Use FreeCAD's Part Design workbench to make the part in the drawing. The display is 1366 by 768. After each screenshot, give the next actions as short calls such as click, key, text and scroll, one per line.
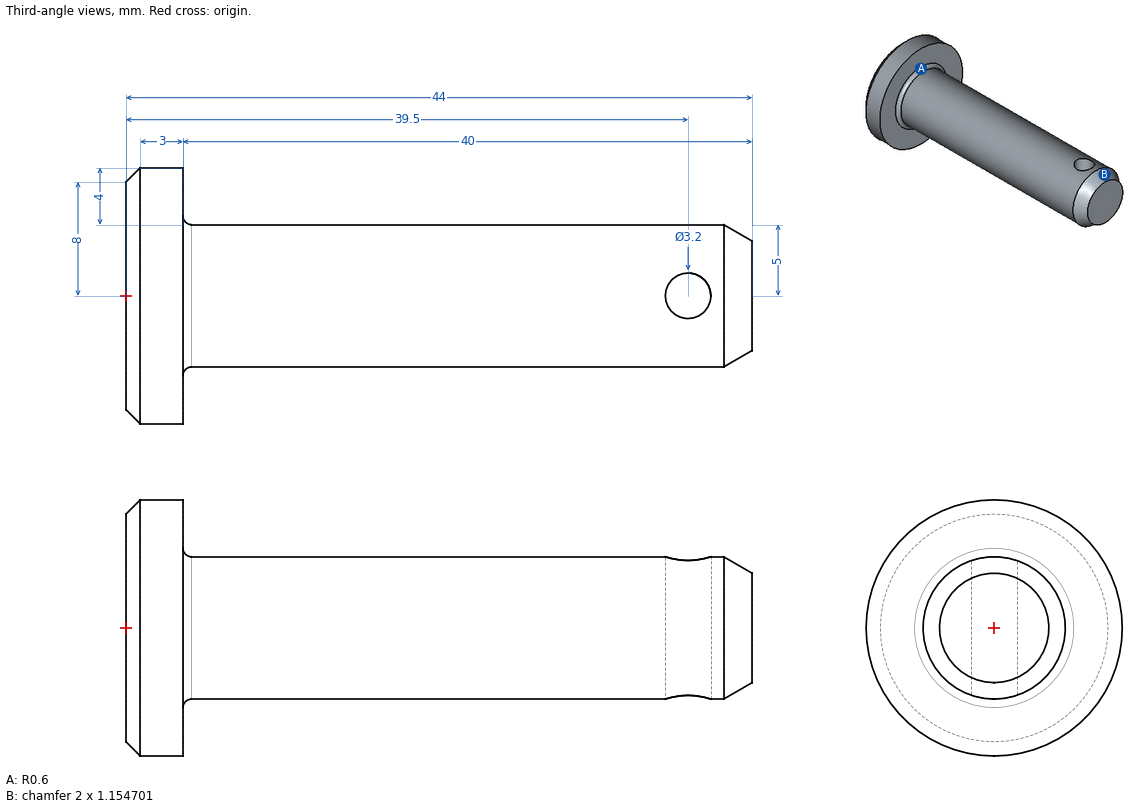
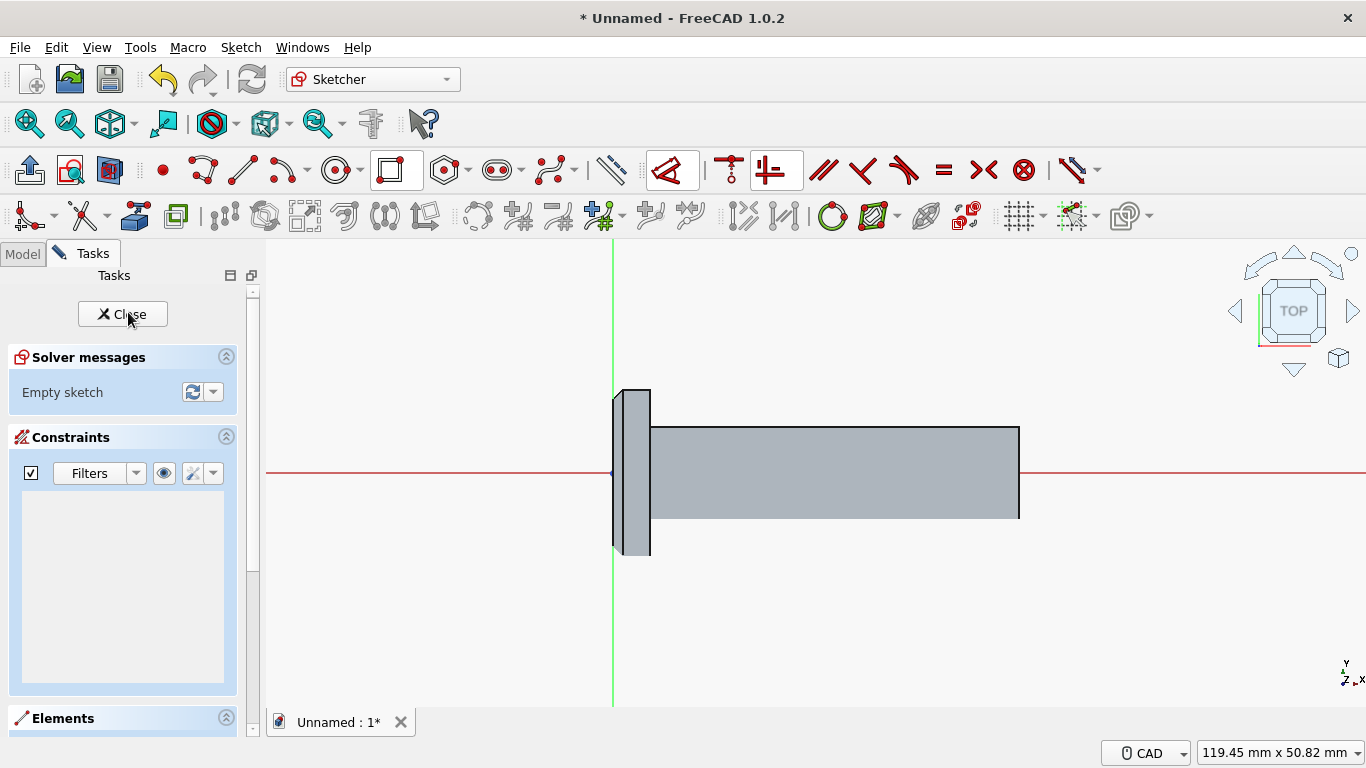
key(q)
key(s)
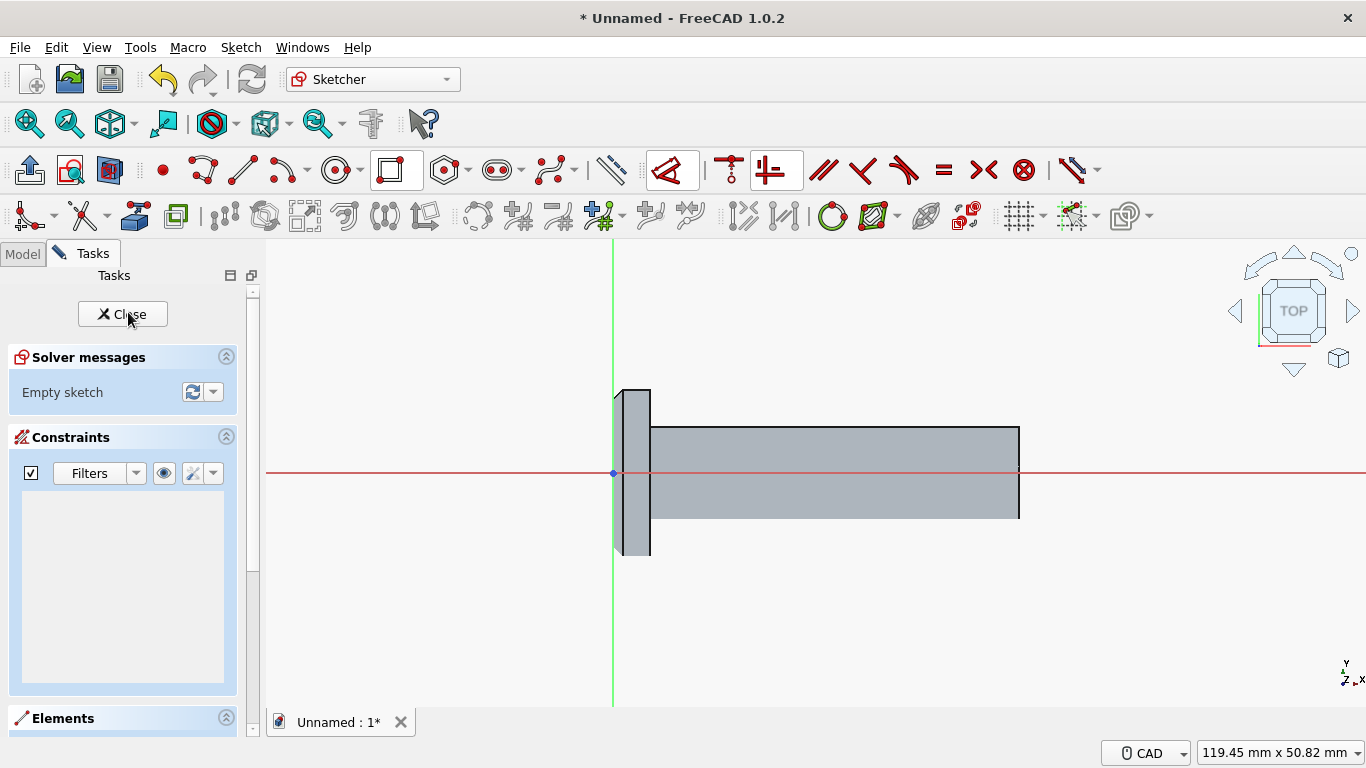
scroll(1006, 473, up, 11)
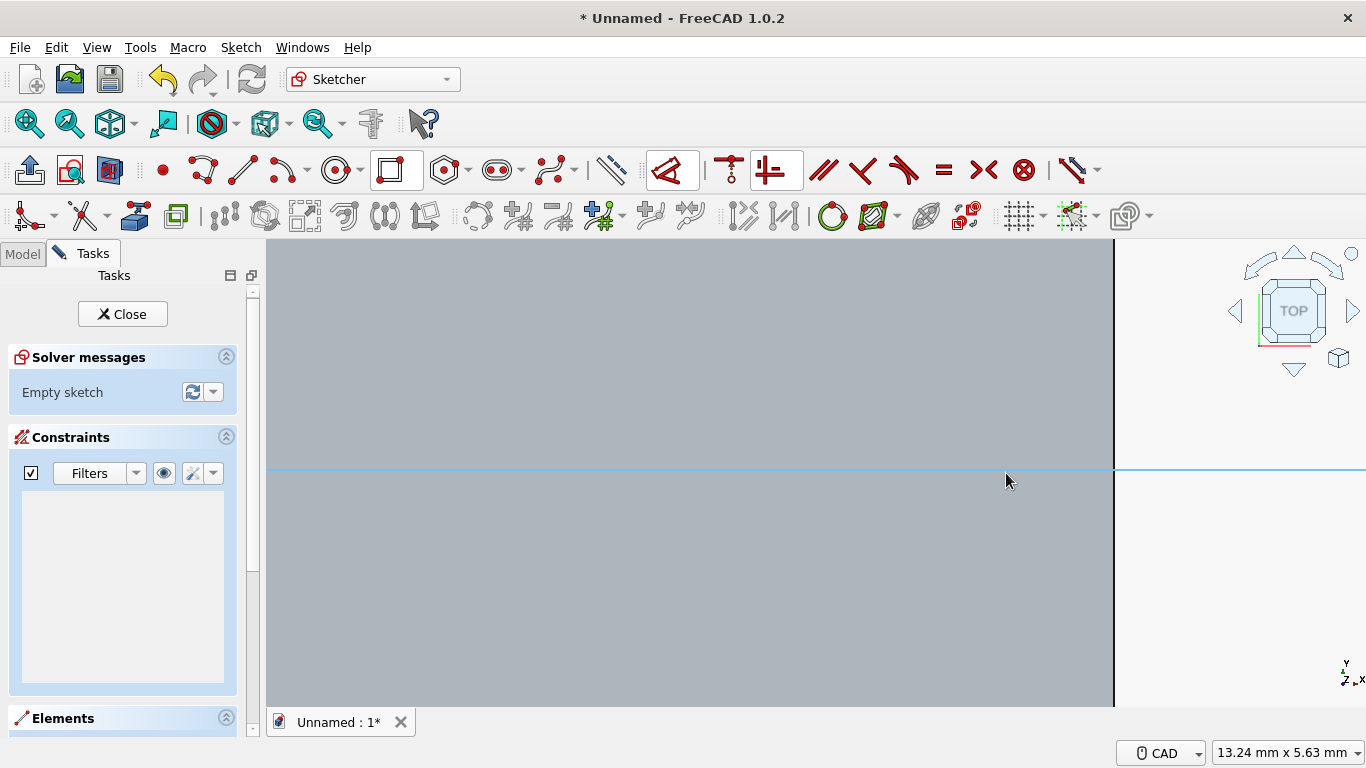
key(g)
key(c)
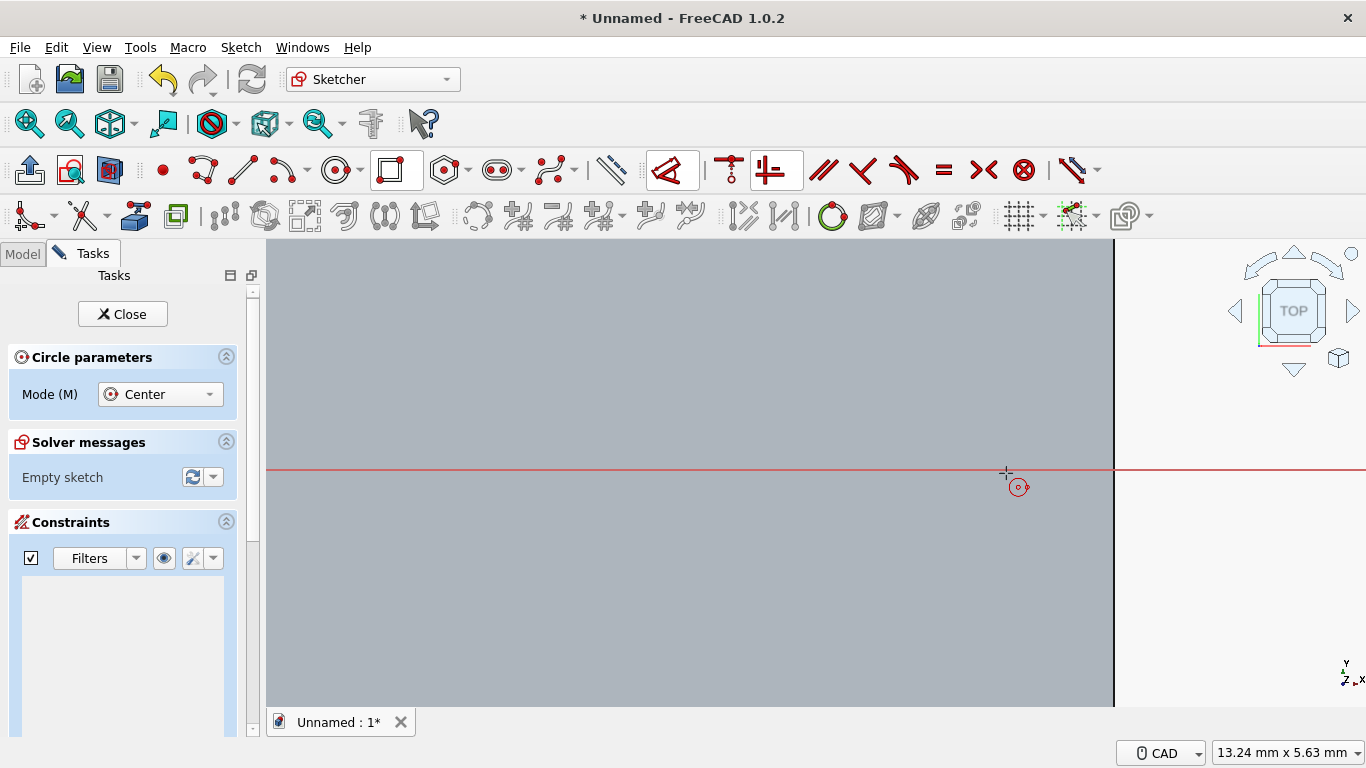
click(740, 470)
move(834, 376)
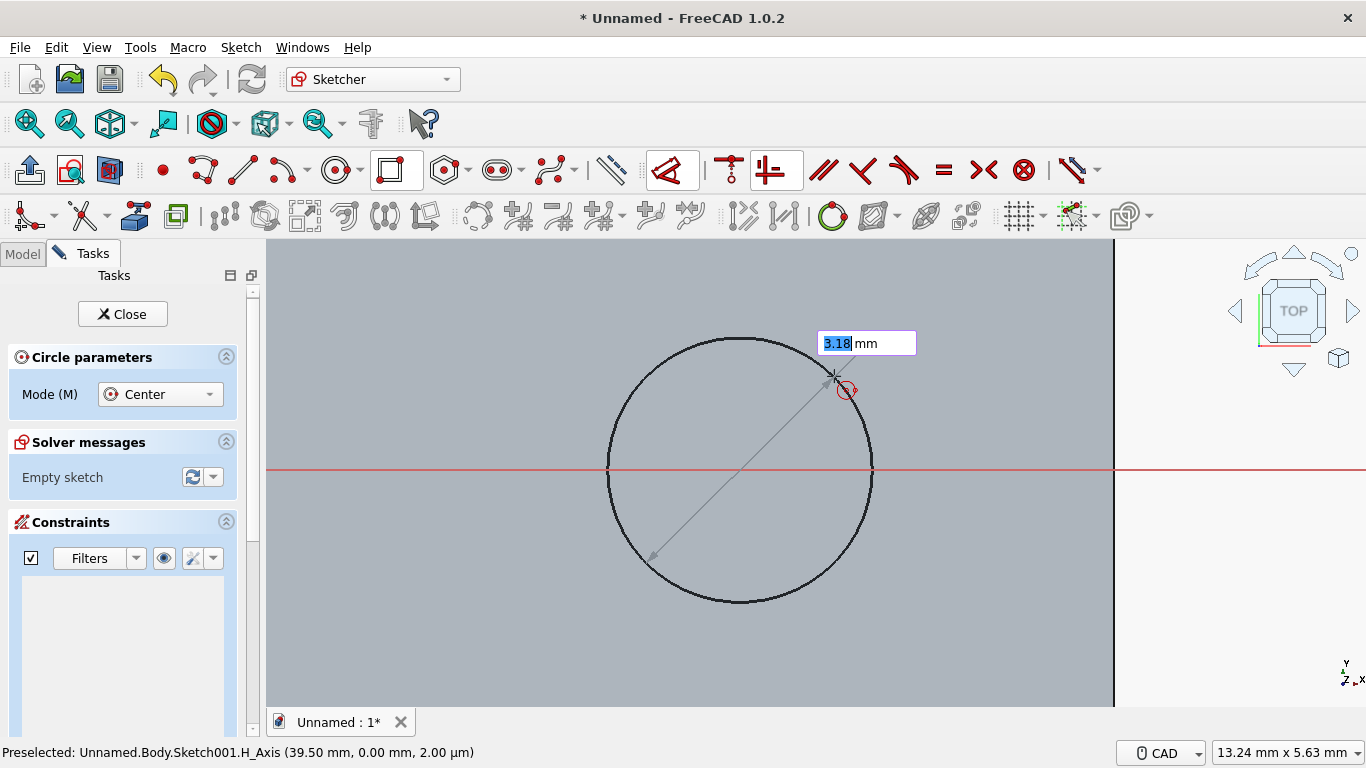
text(3.2)
key(Return)
key(Escape)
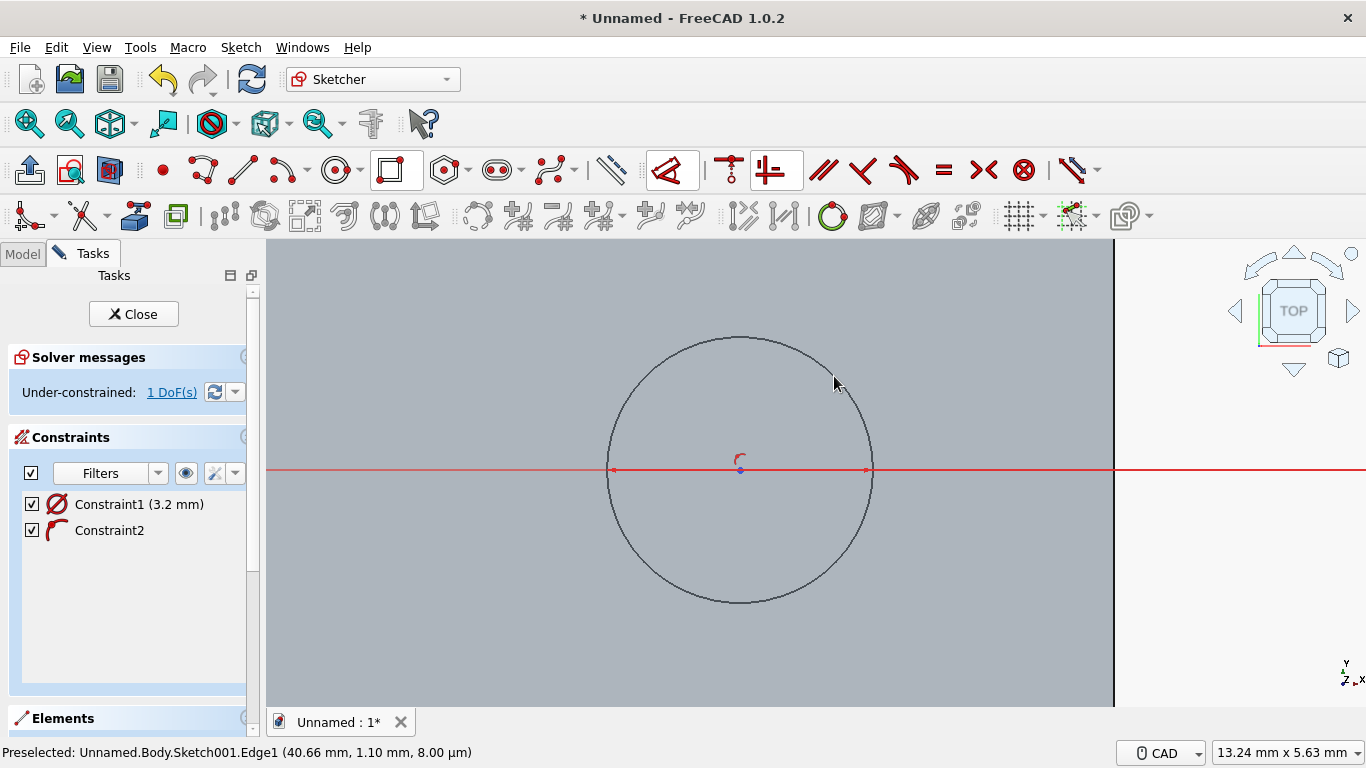
click(740, 470)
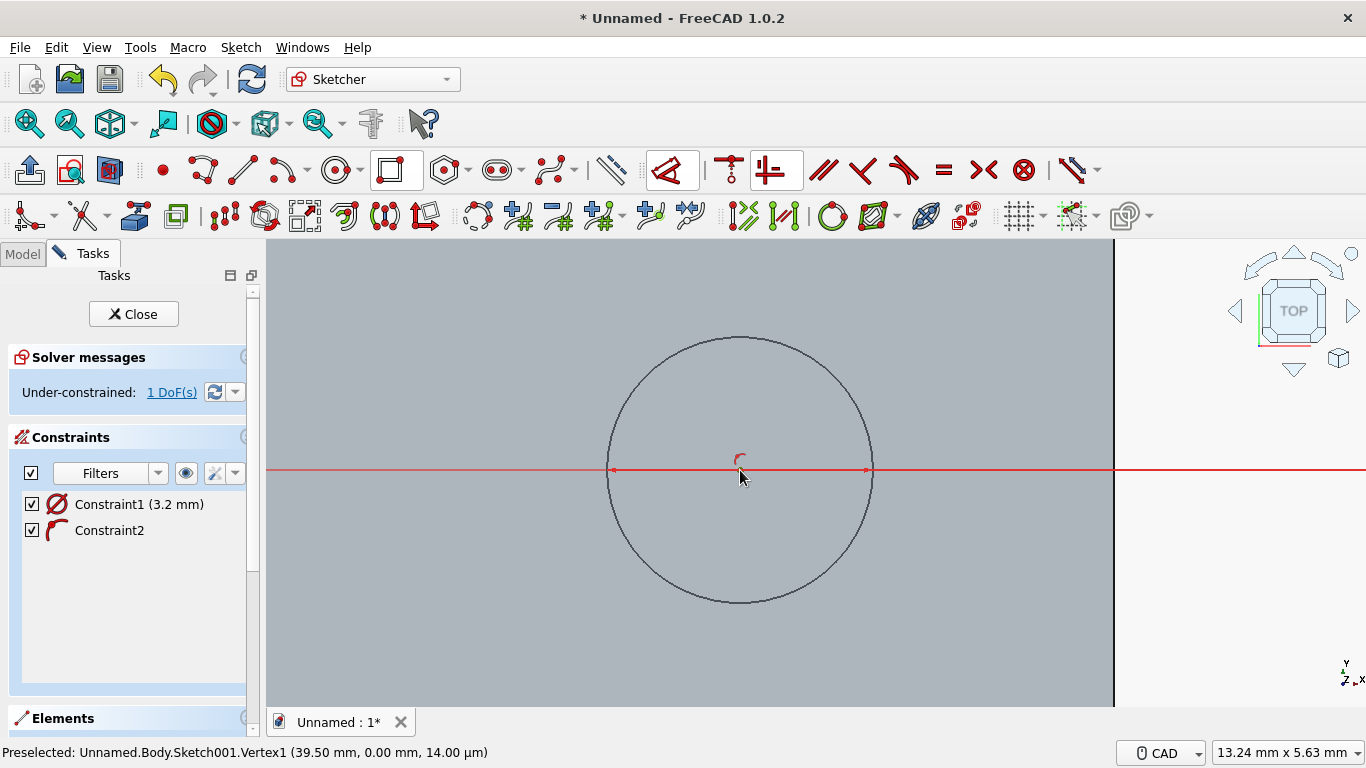
key(l)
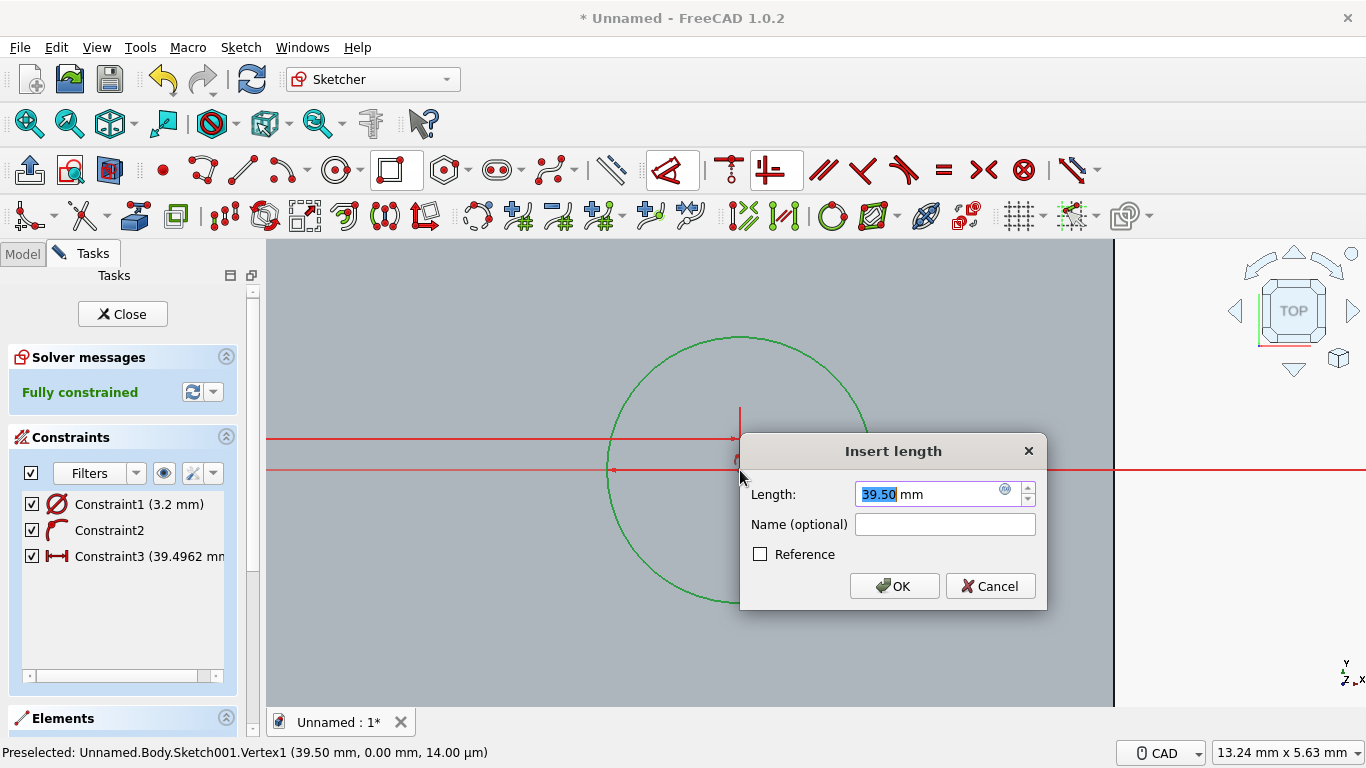
text(39.5)
key(Return)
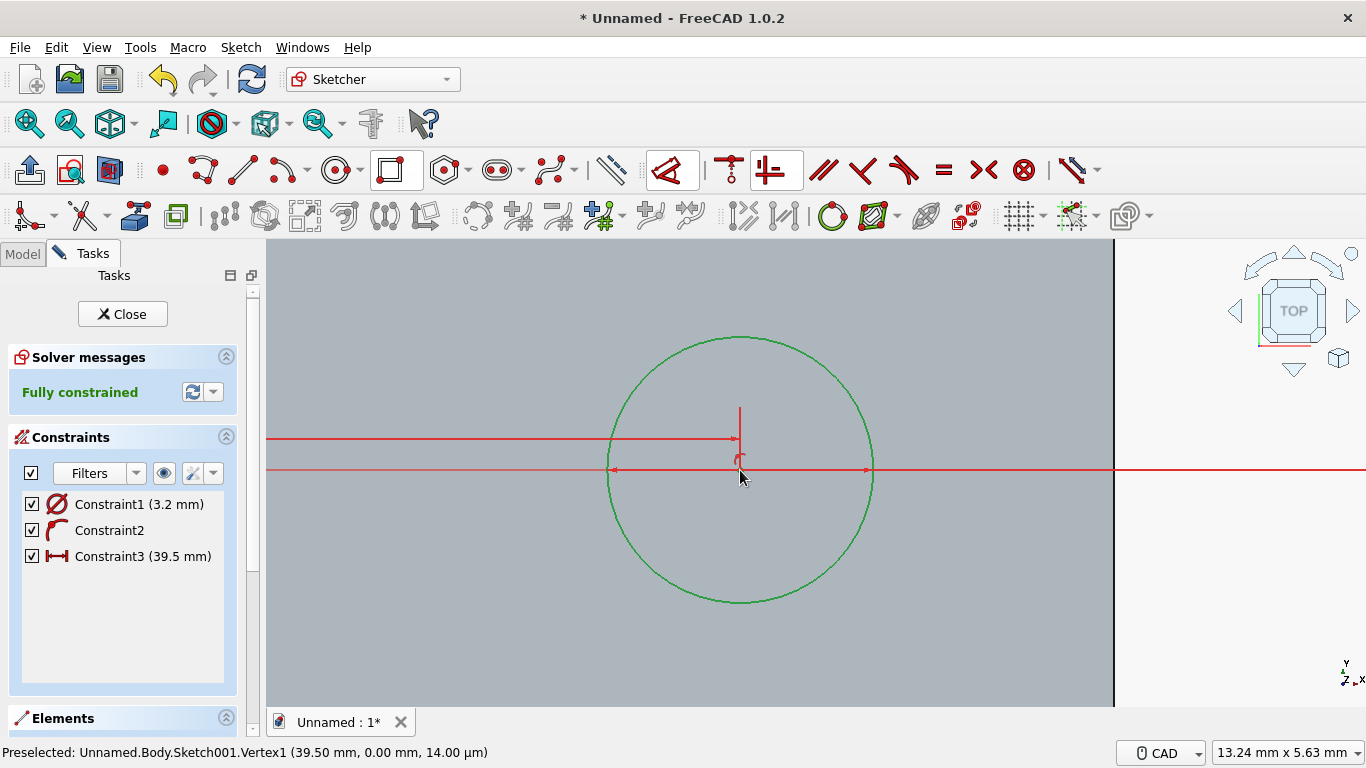
click(123, 314)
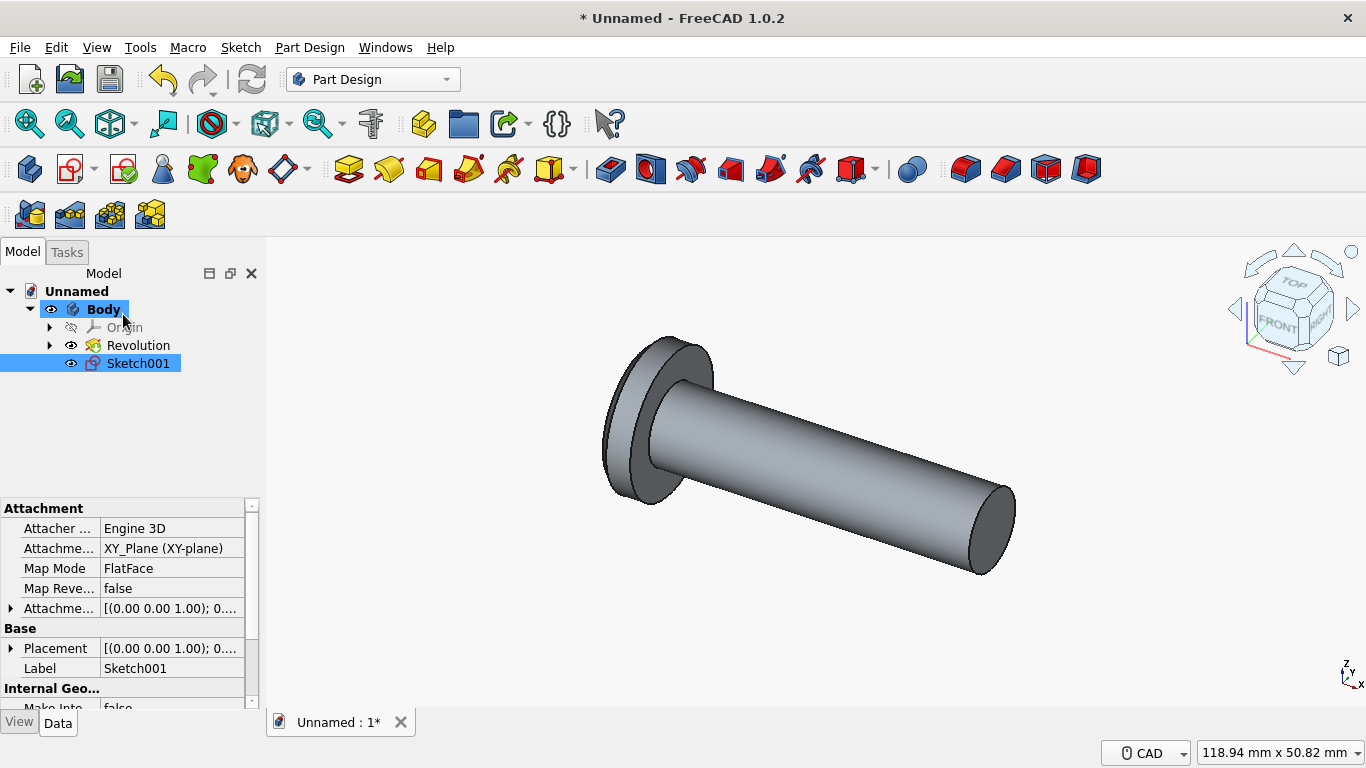
click(612, 170)